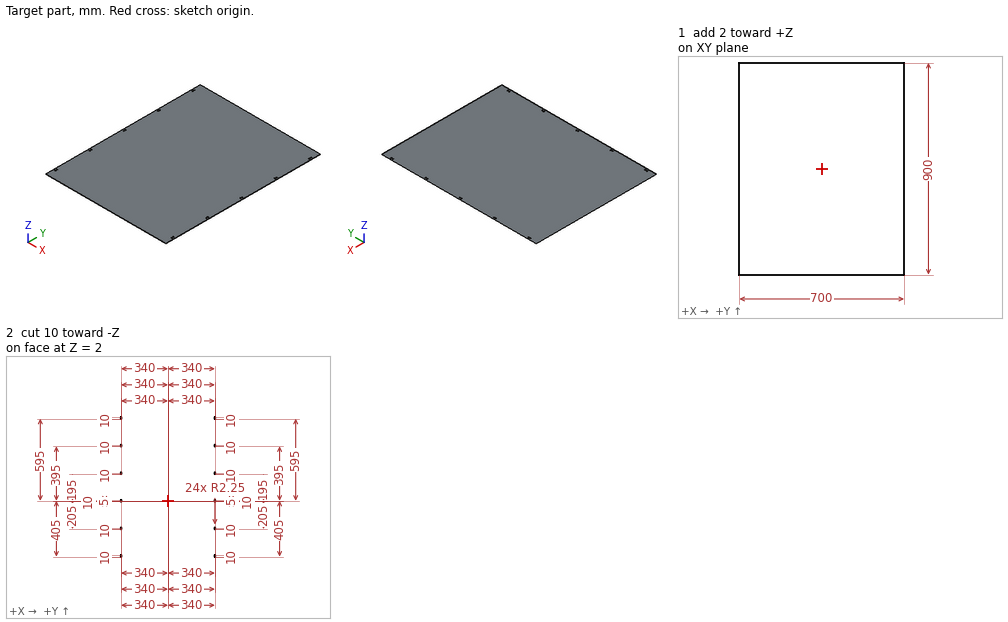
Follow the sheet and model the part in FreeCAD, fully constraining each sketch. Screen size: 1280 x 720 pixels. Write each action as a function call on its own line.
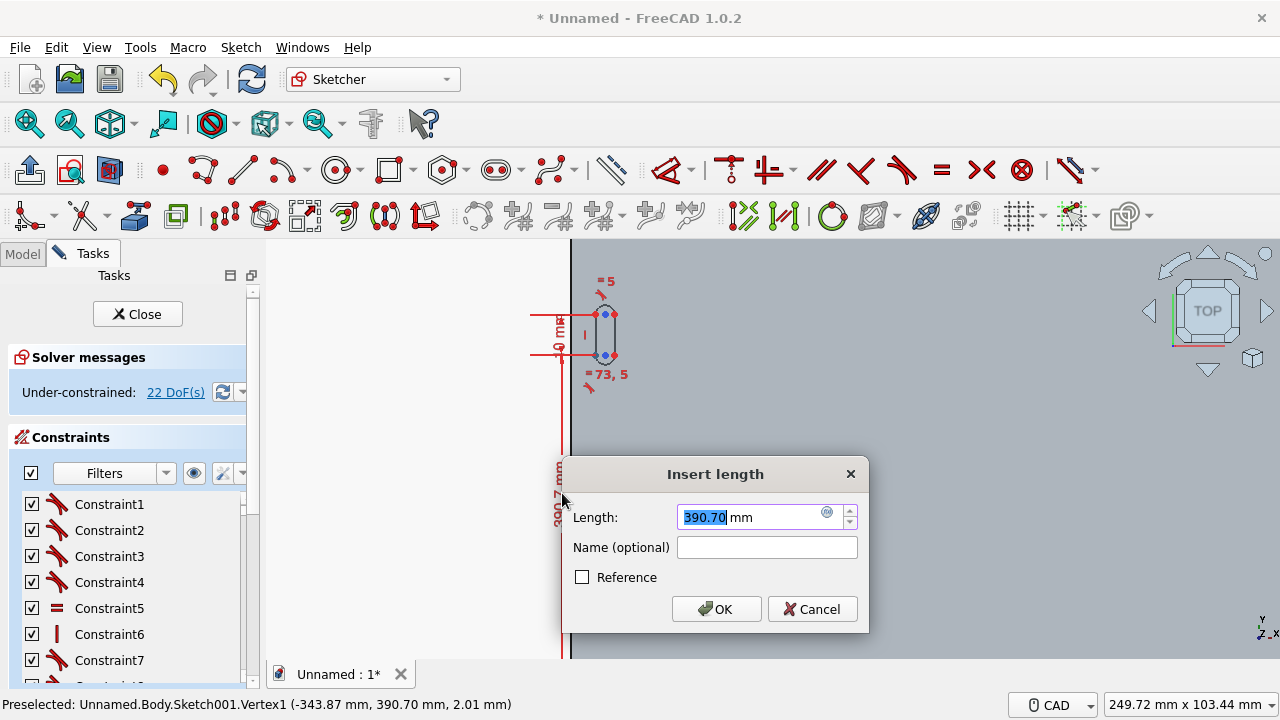
text(395)
key(Return)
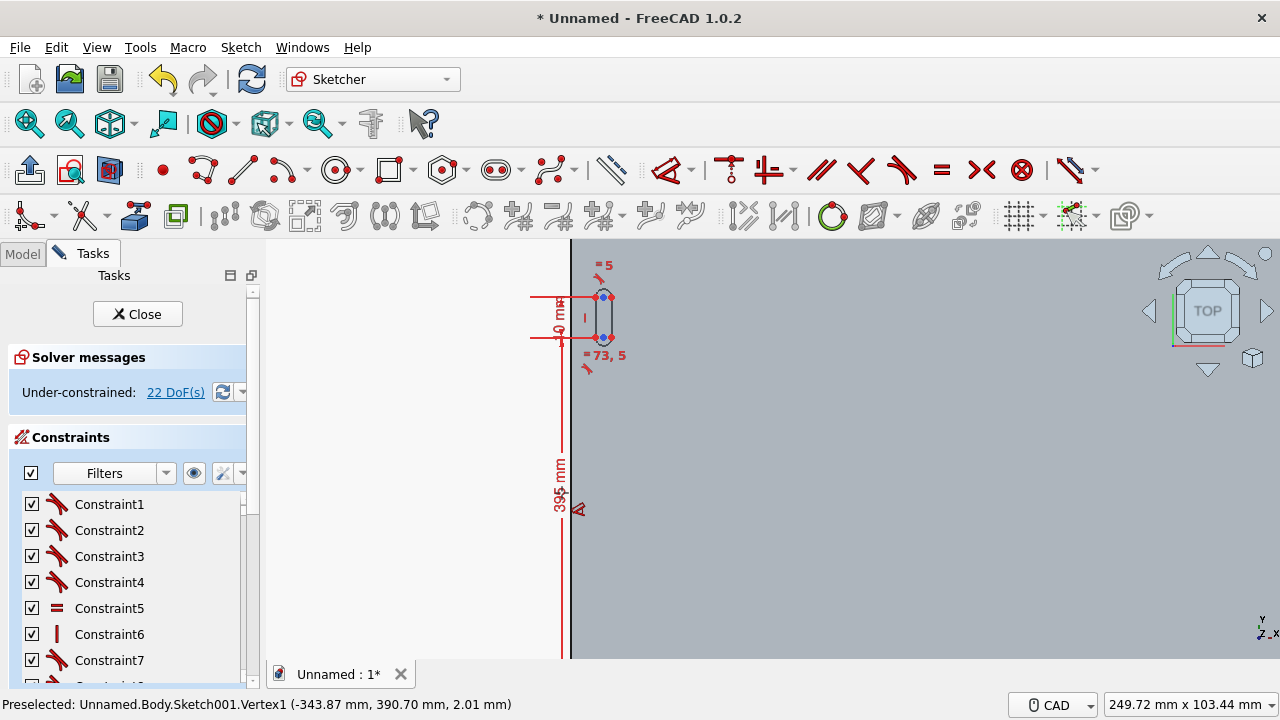
scroll(621, 379, down, 14)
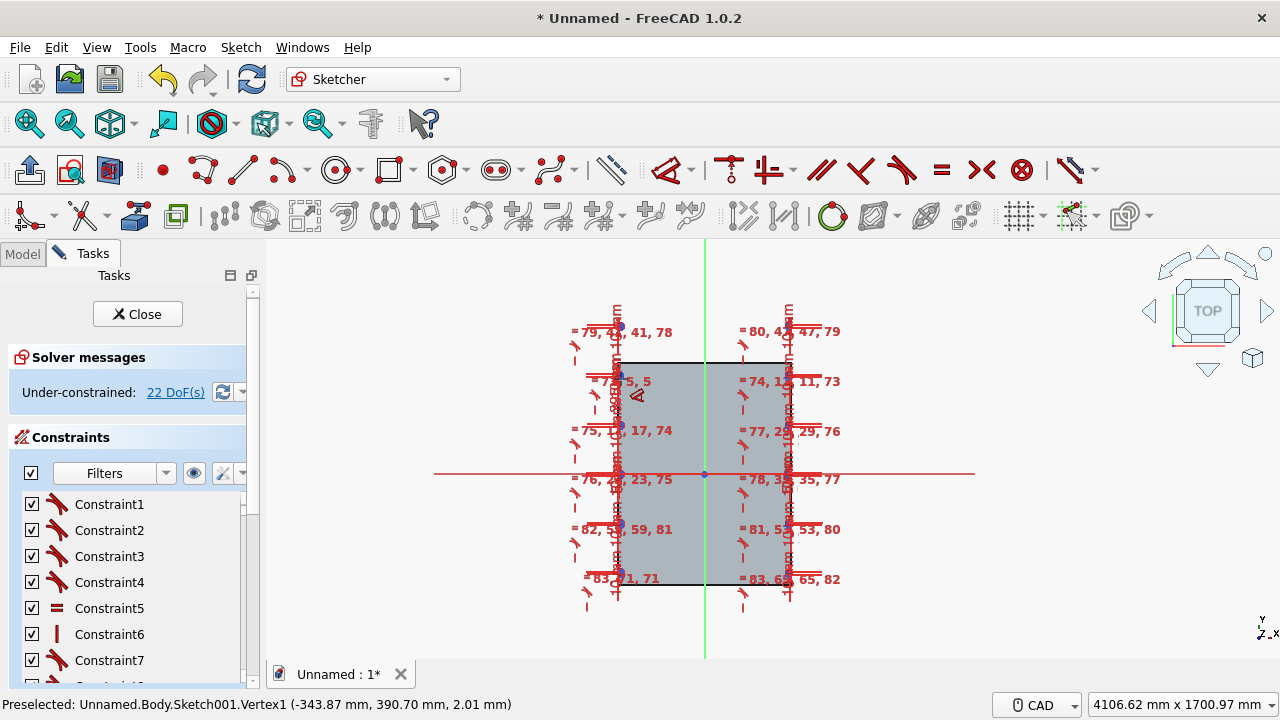
scroll(788, 377, up, 14)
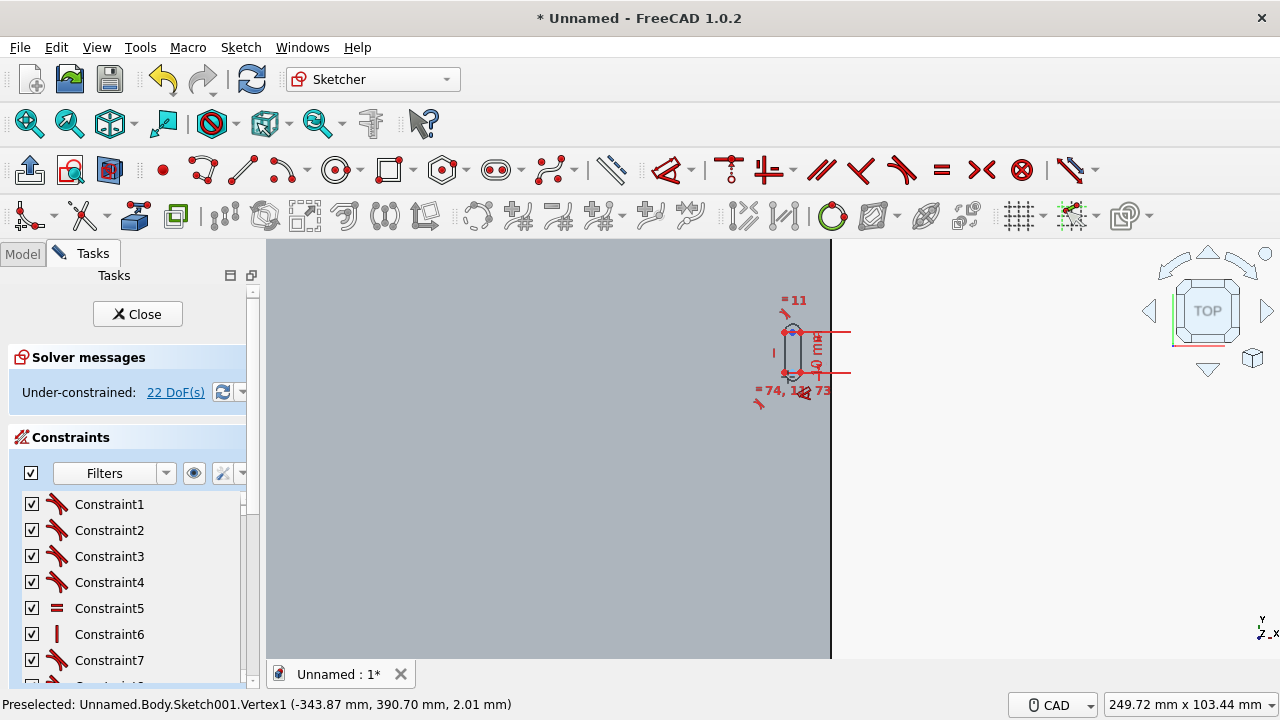
click(785, 373)
click(819, 502)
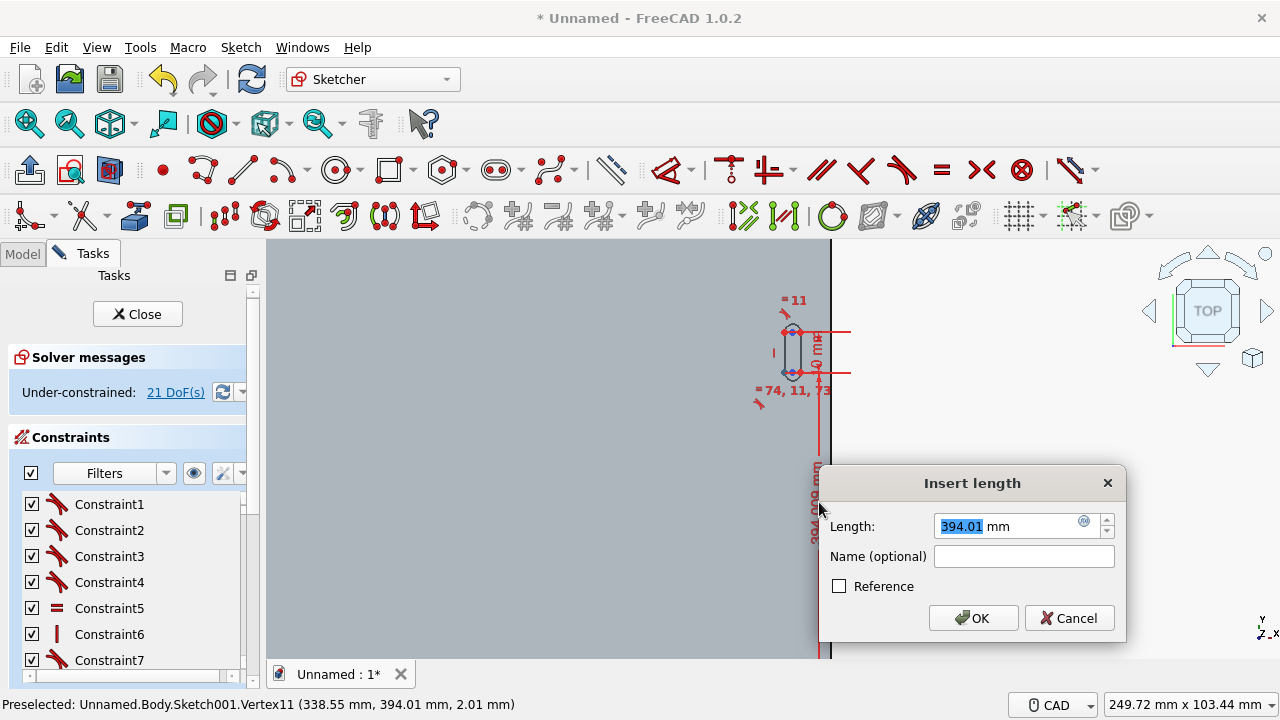
text(395)
key(Return)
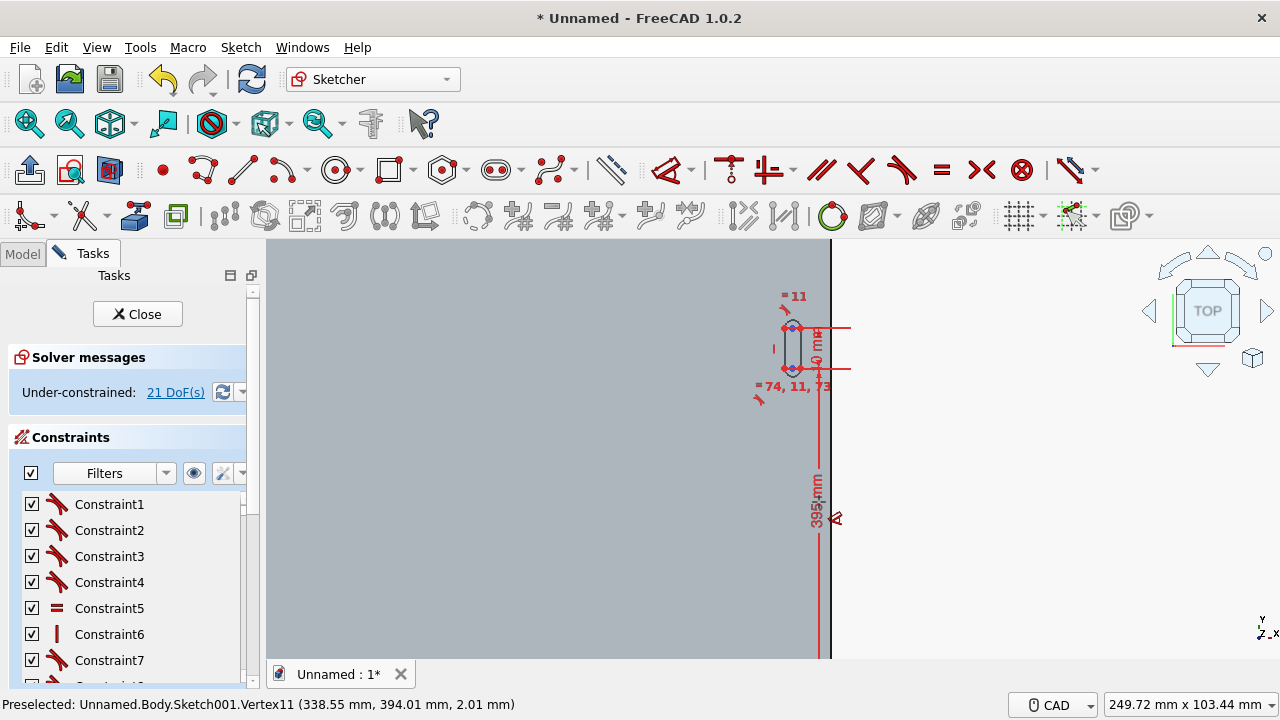
scroll(788, 377, down, 14)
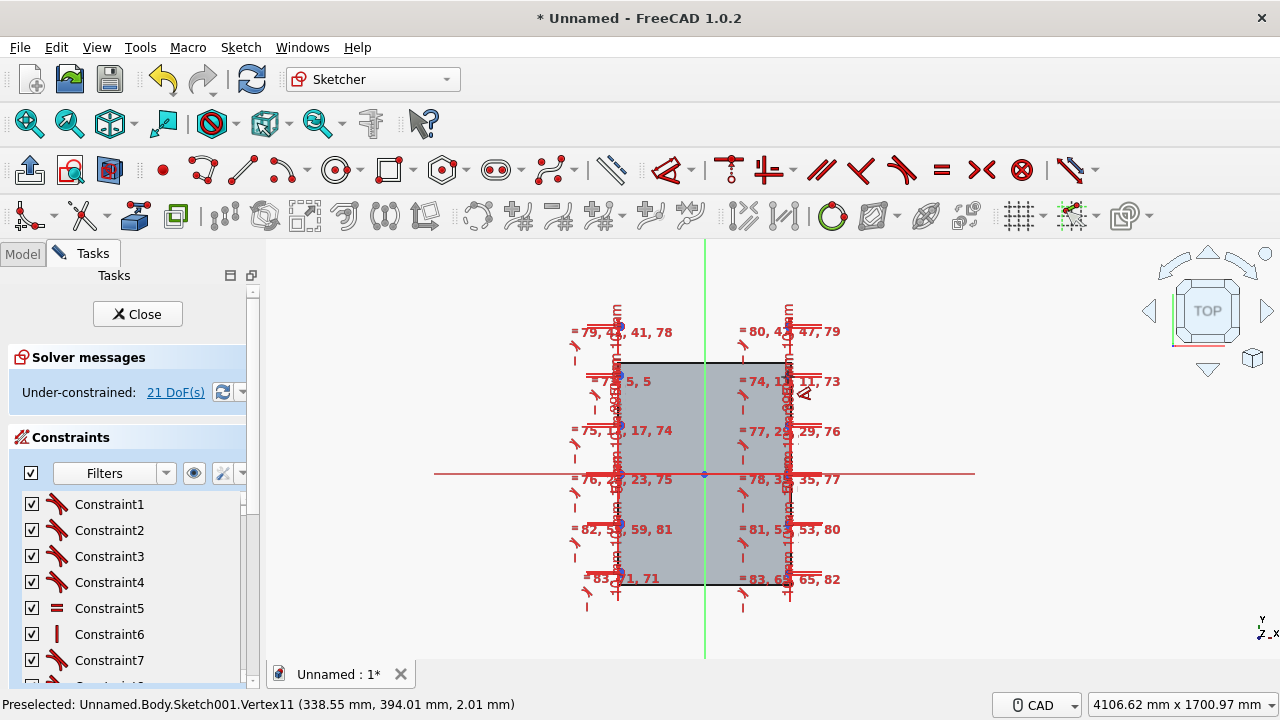
scroll(621, 427, up, 14)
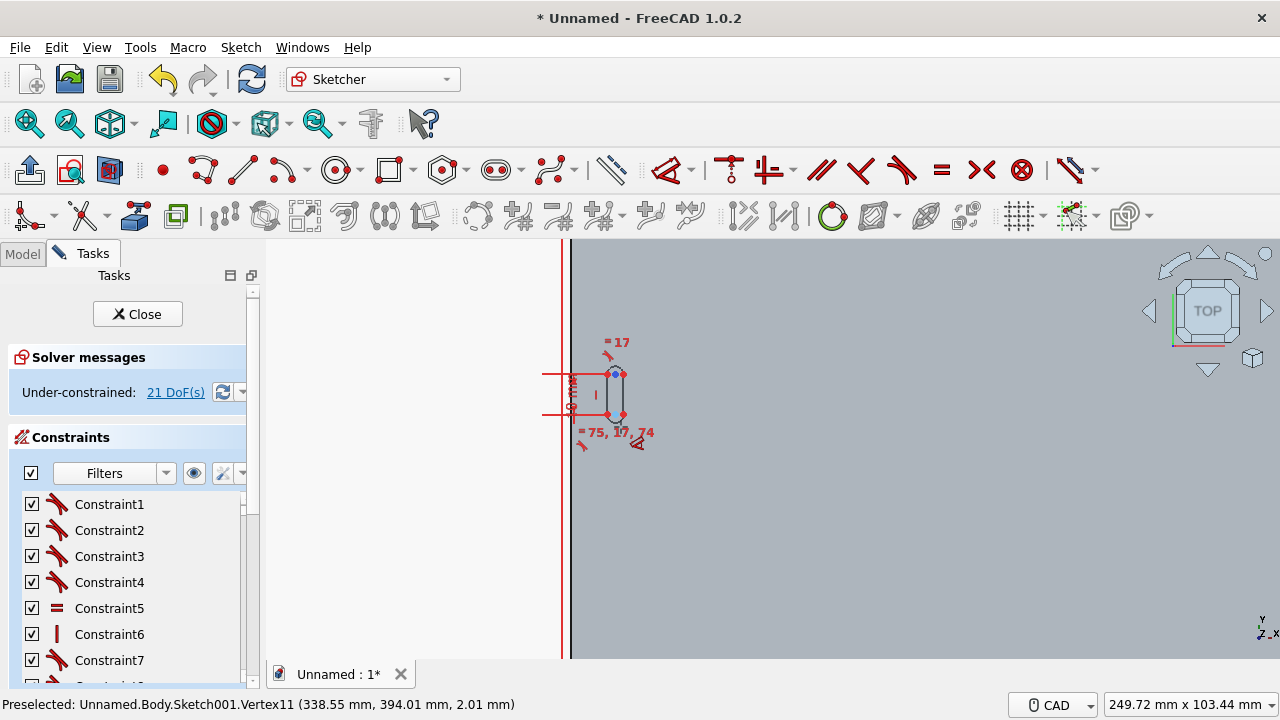
click(607, 415)
click(573, 523)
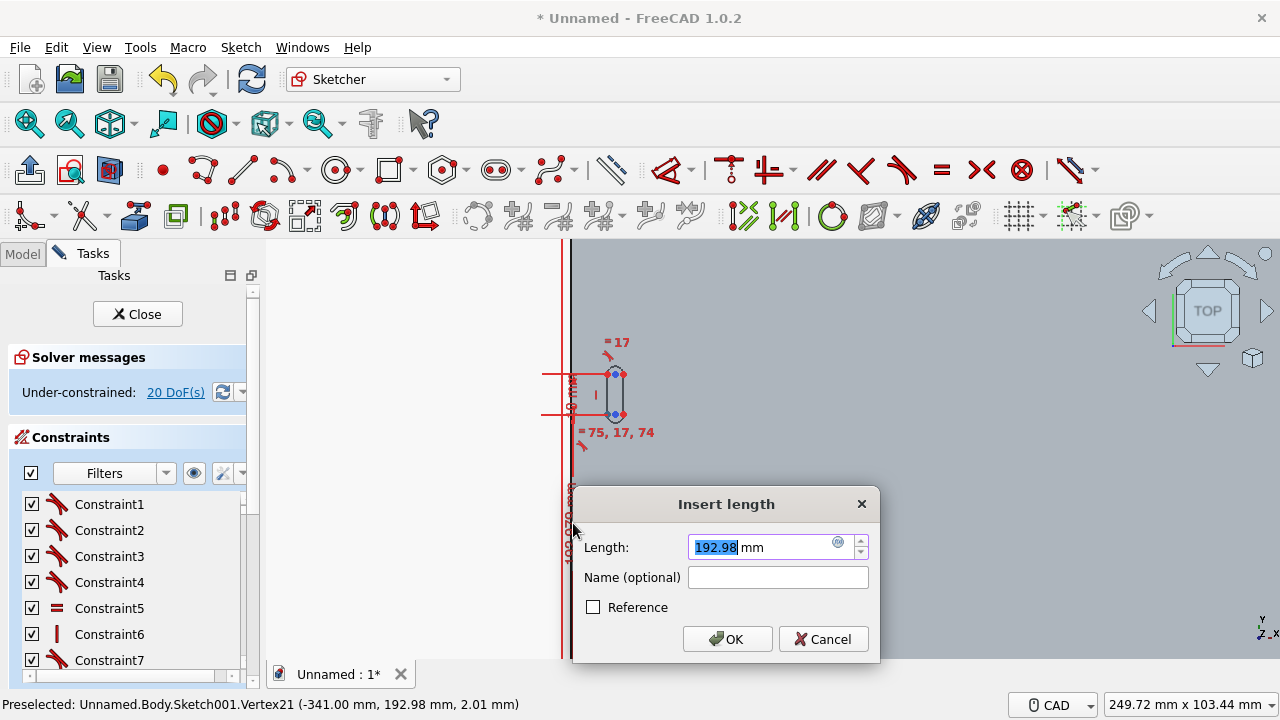
text(195)
key(Return)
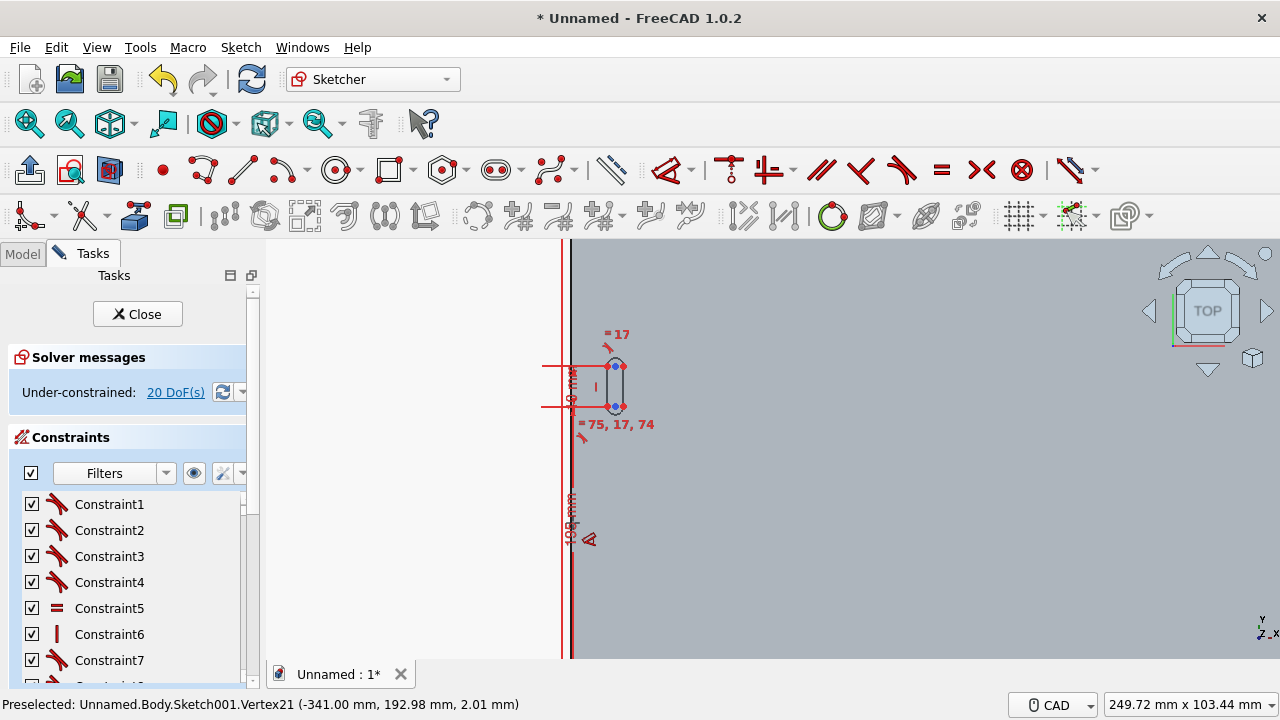
scroll(621, 427, down, 14)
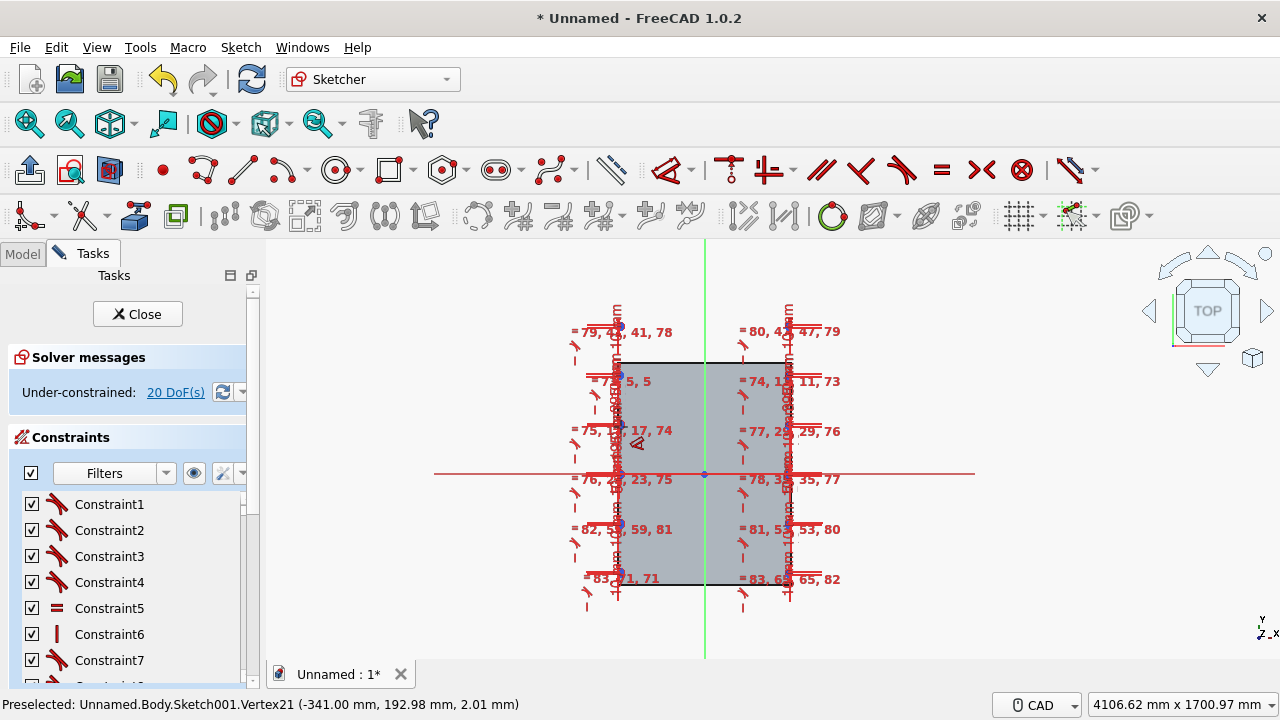
scroll(788, 427, up, 14)